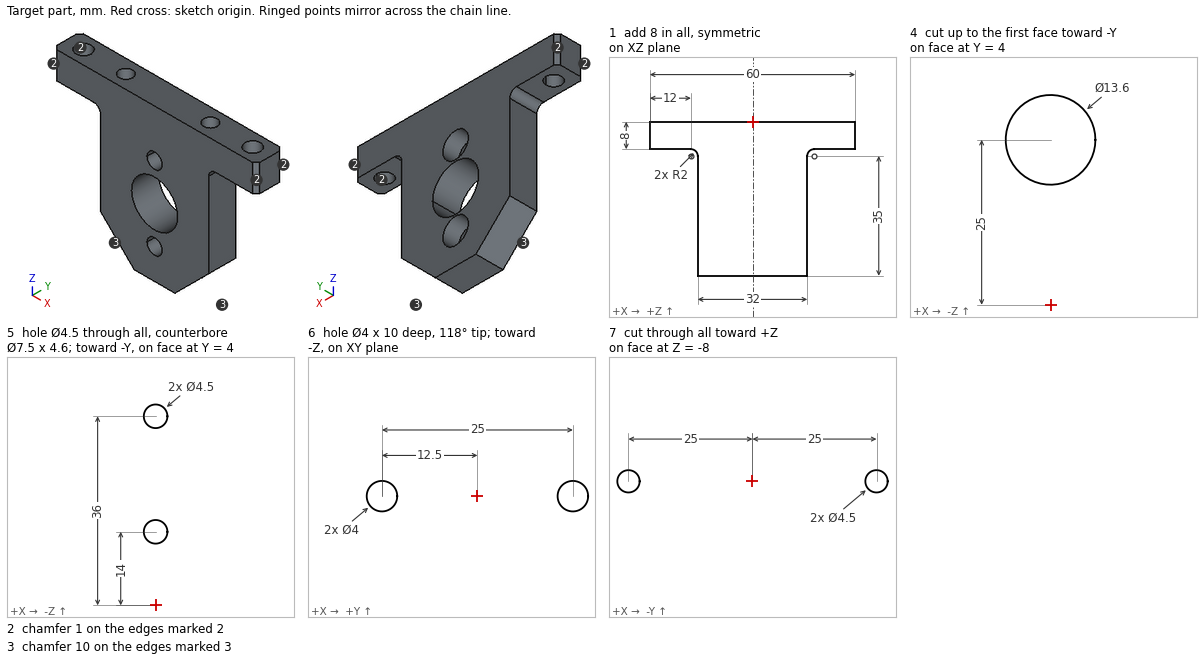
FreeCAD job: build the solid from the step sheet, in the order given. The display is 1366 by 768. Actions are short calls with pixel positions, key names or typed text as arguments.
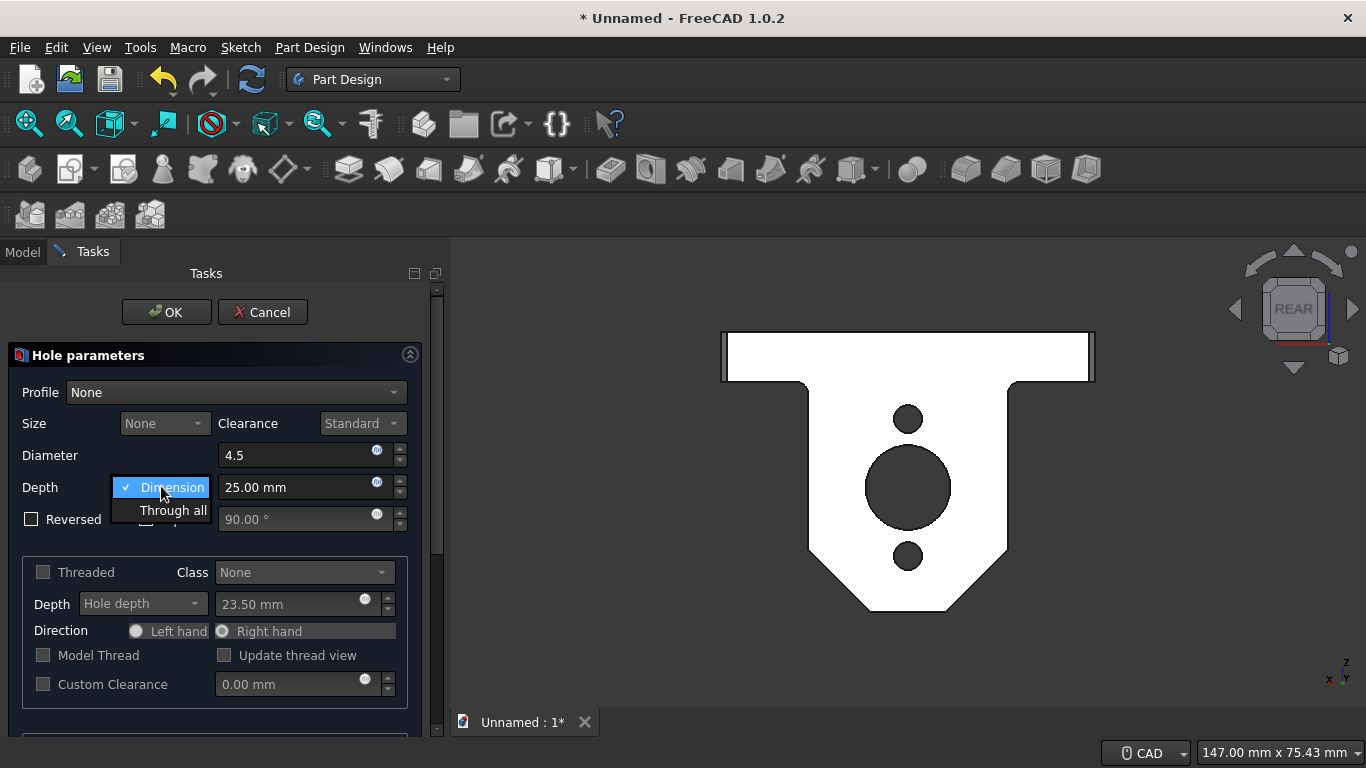
click(160, 510)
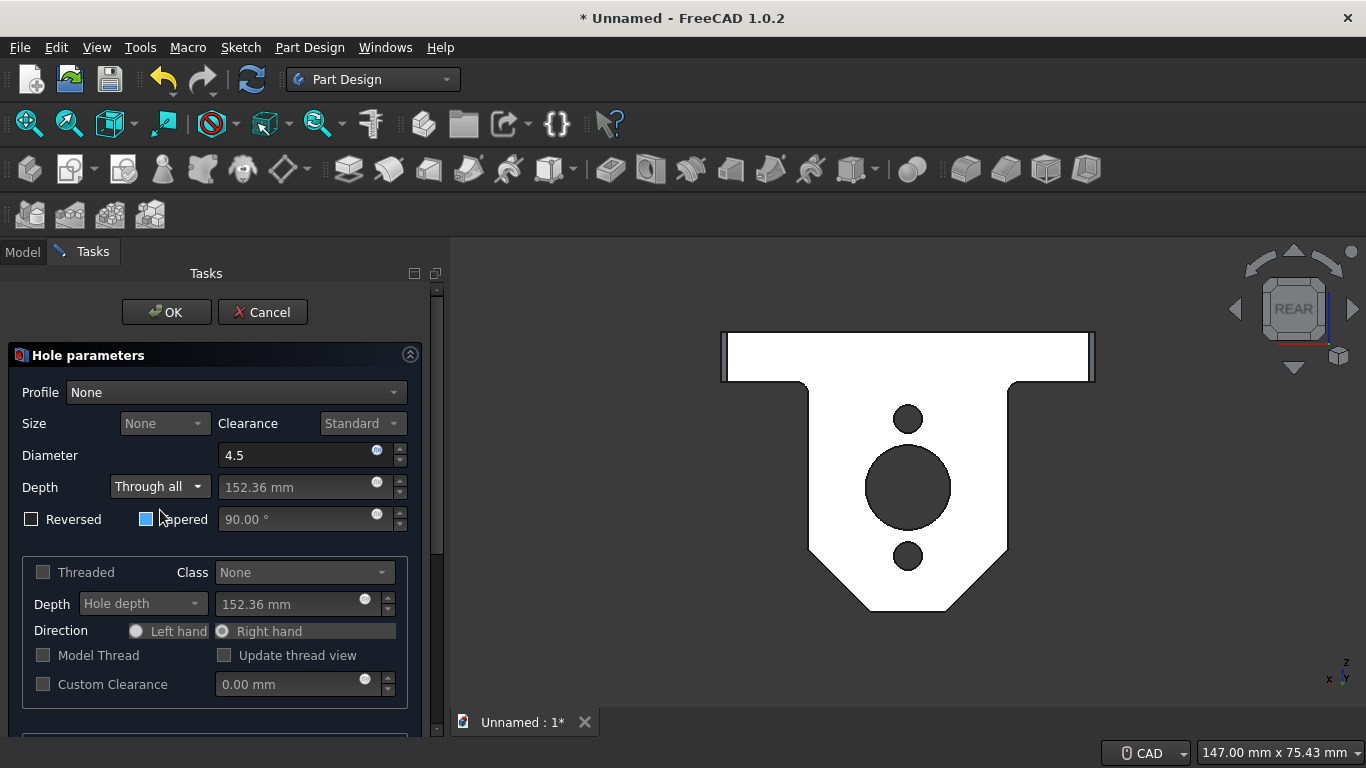
scroll(437, 510, down, 2)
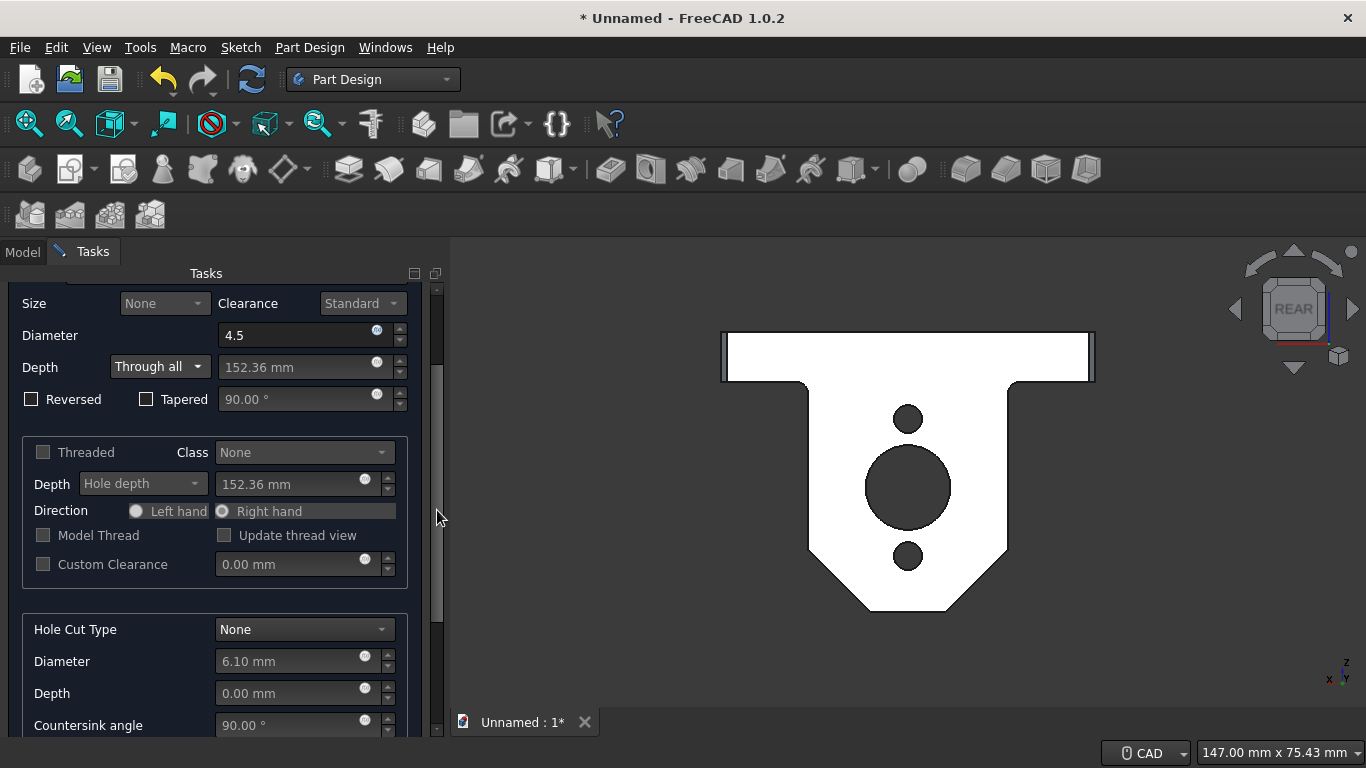
click(306, 630)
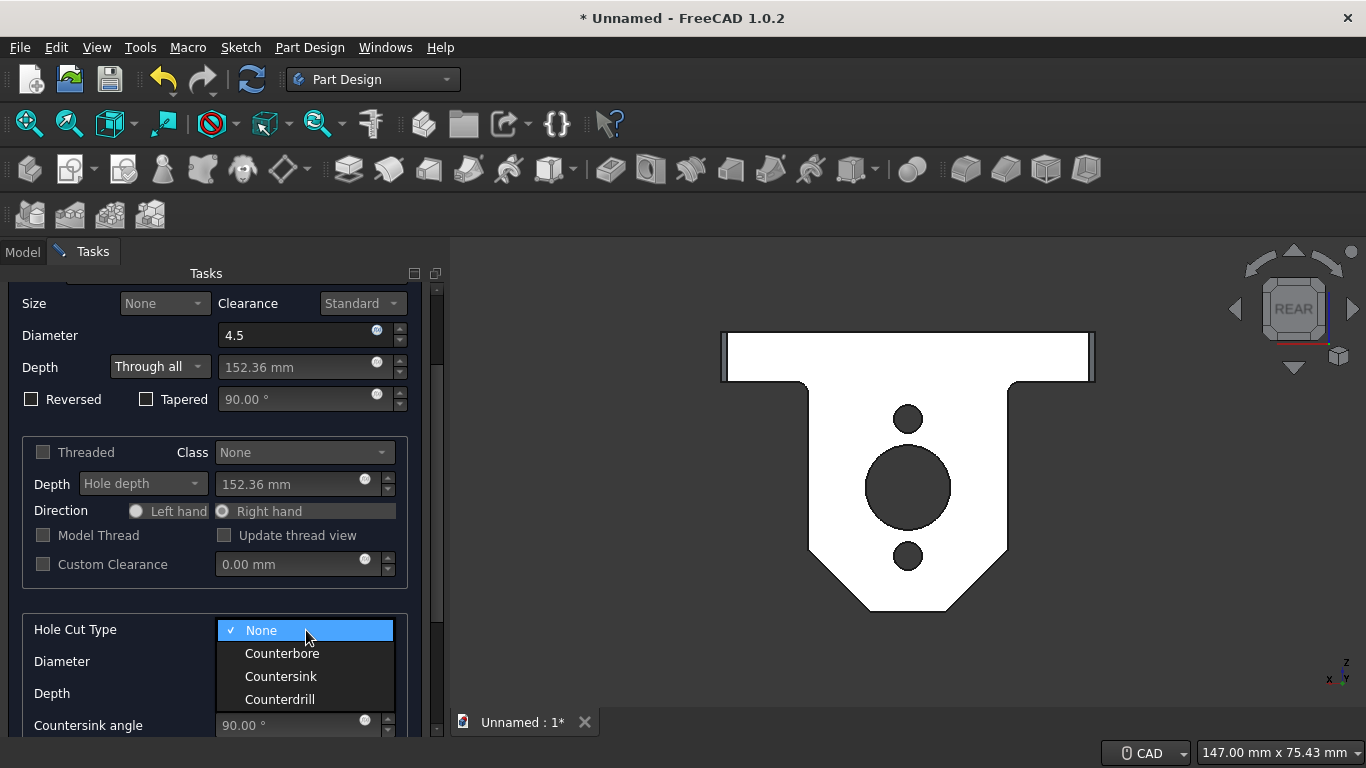
click(304, 654)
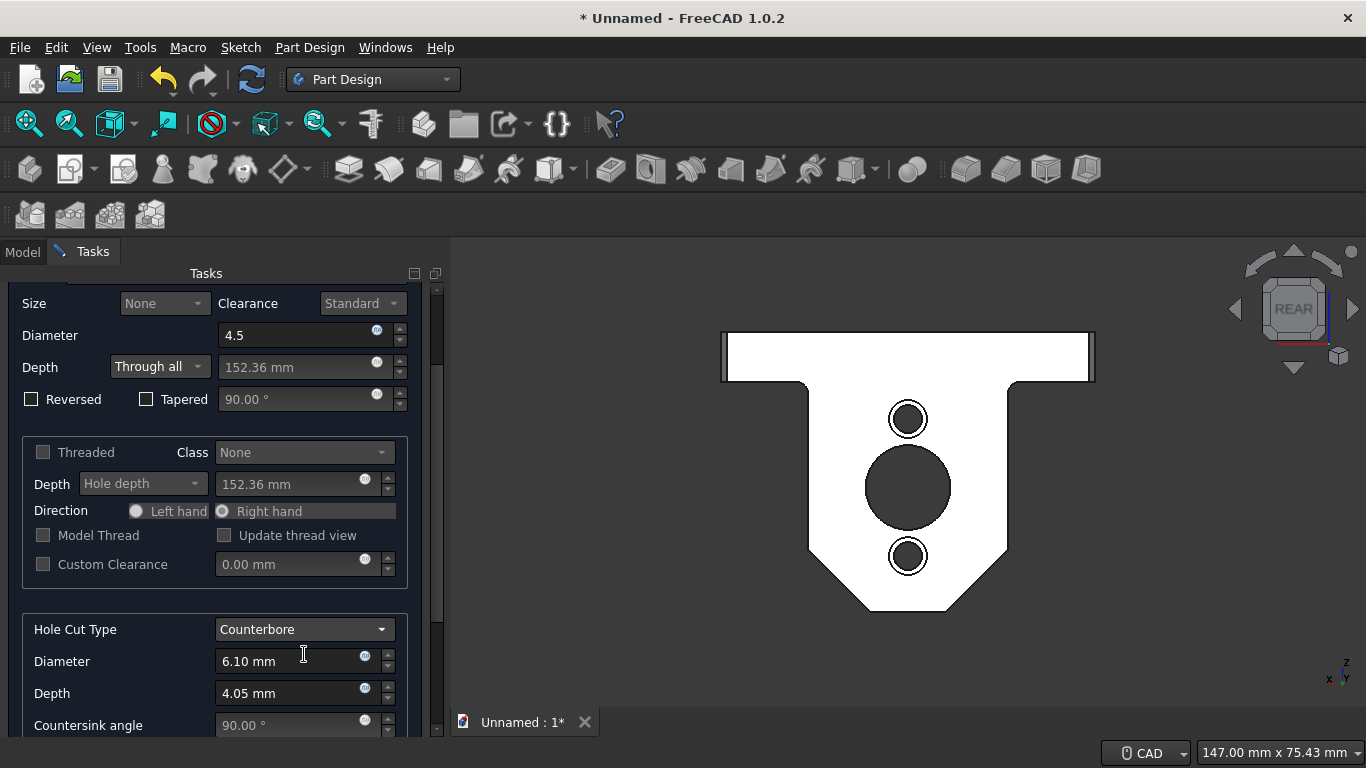
triple_click(298, 661)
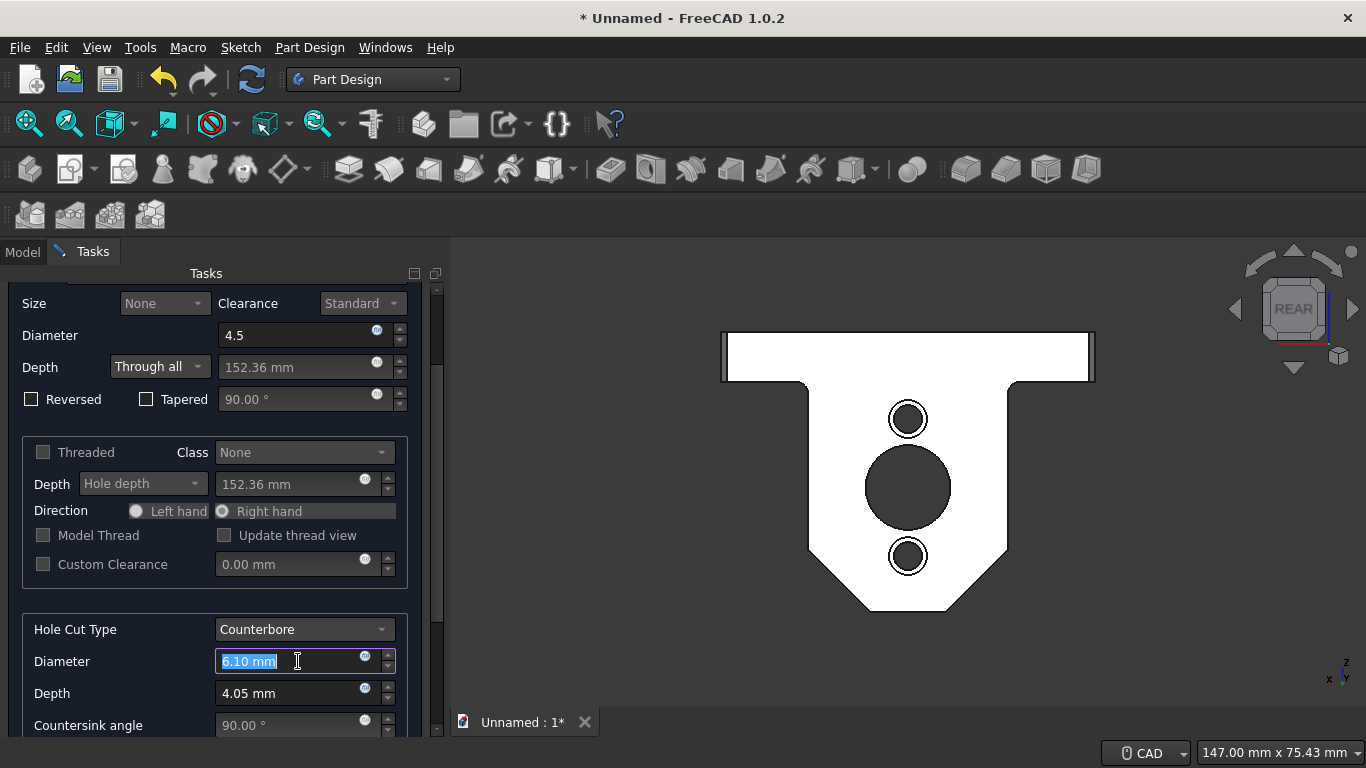
text(7.5)
key(Tab)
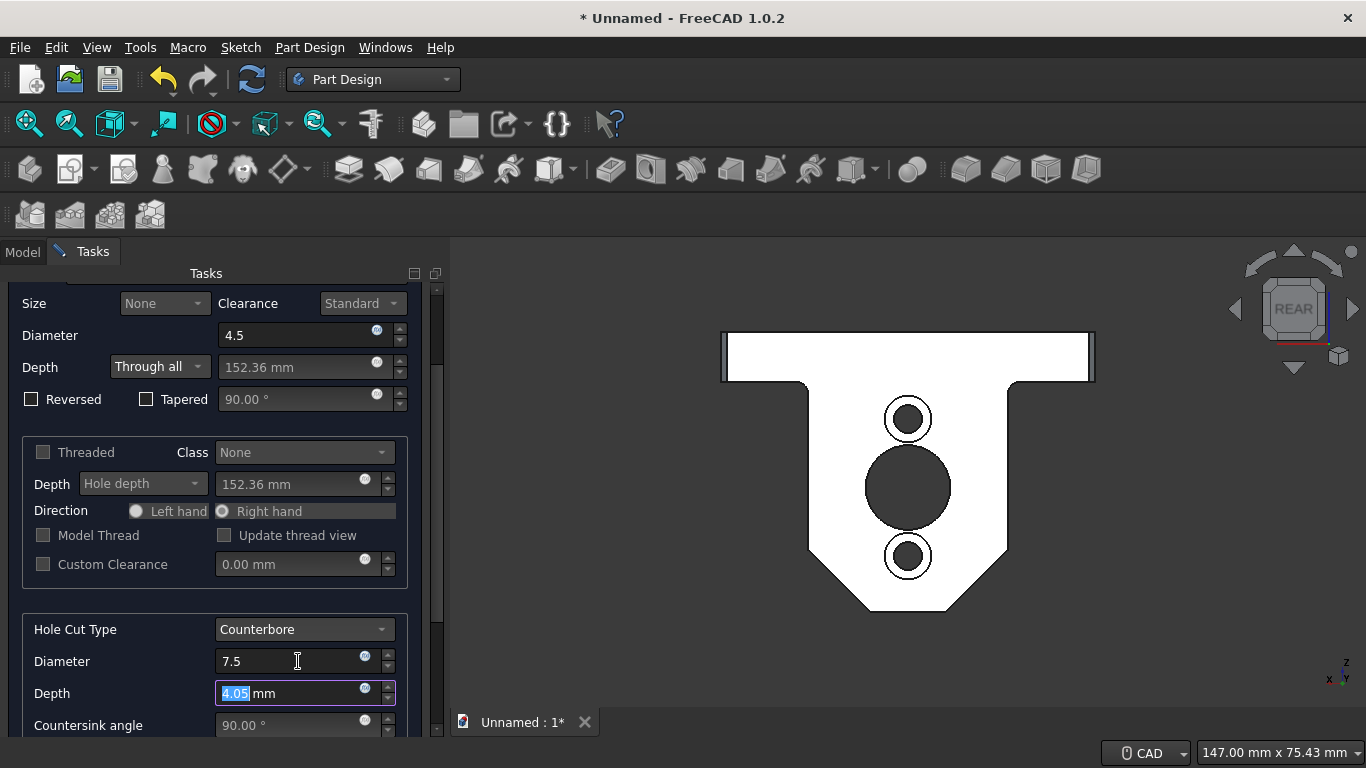
text(4.6)
key(Tab)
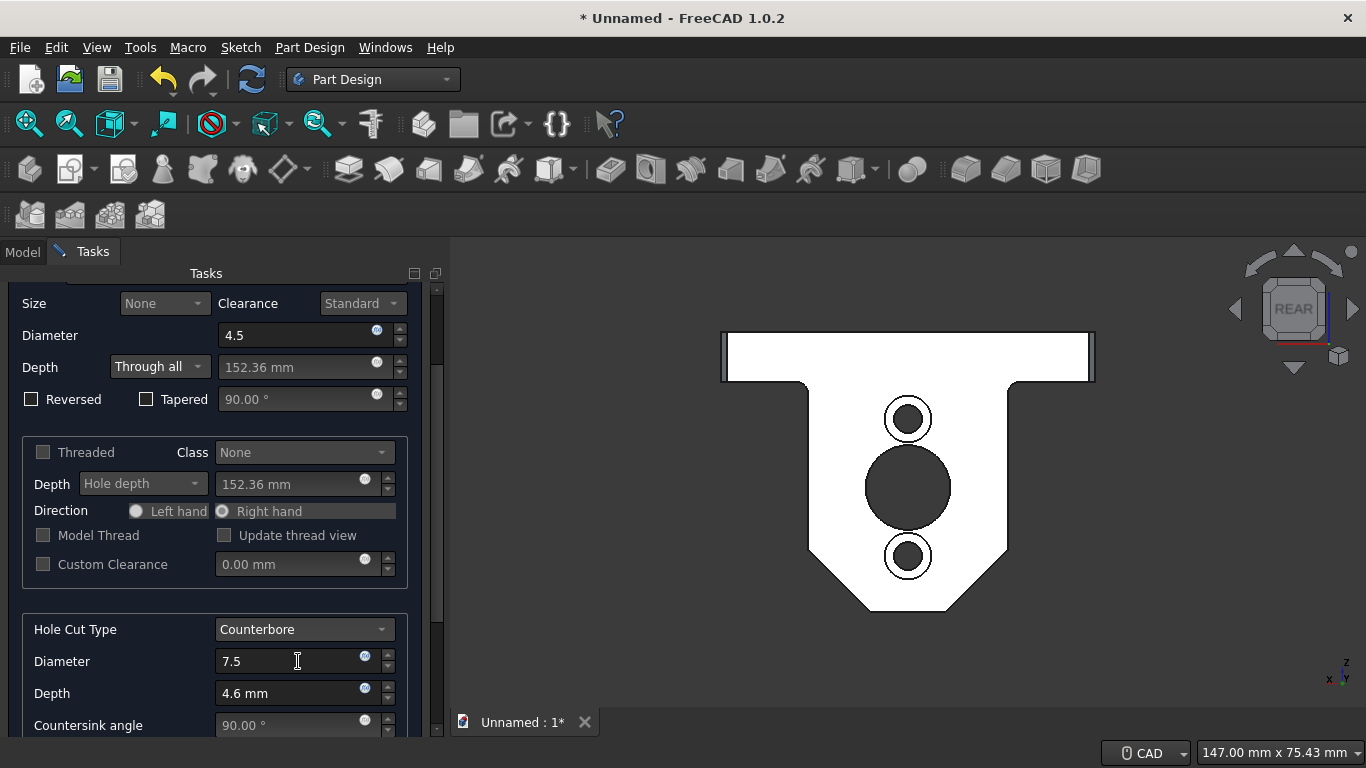
scroll(437, 510, up, 3)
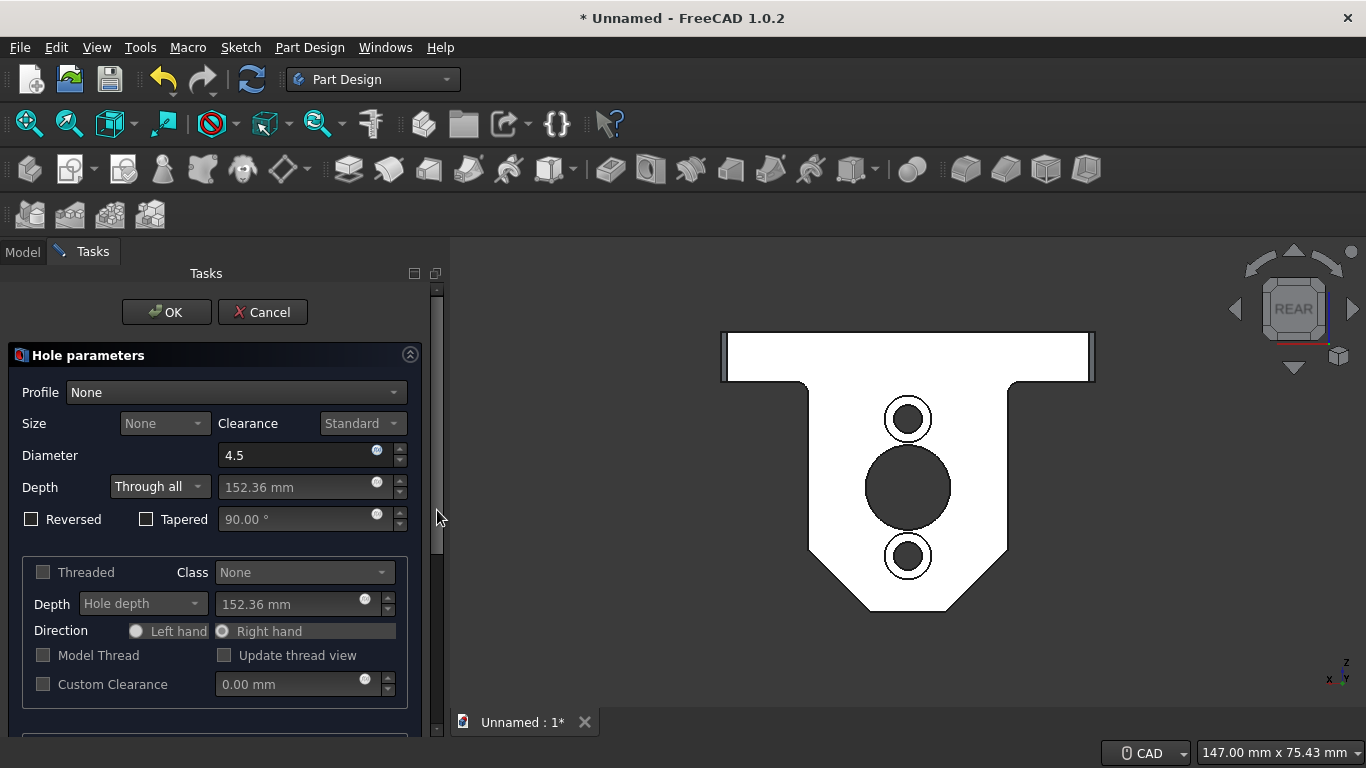
click(167, 312)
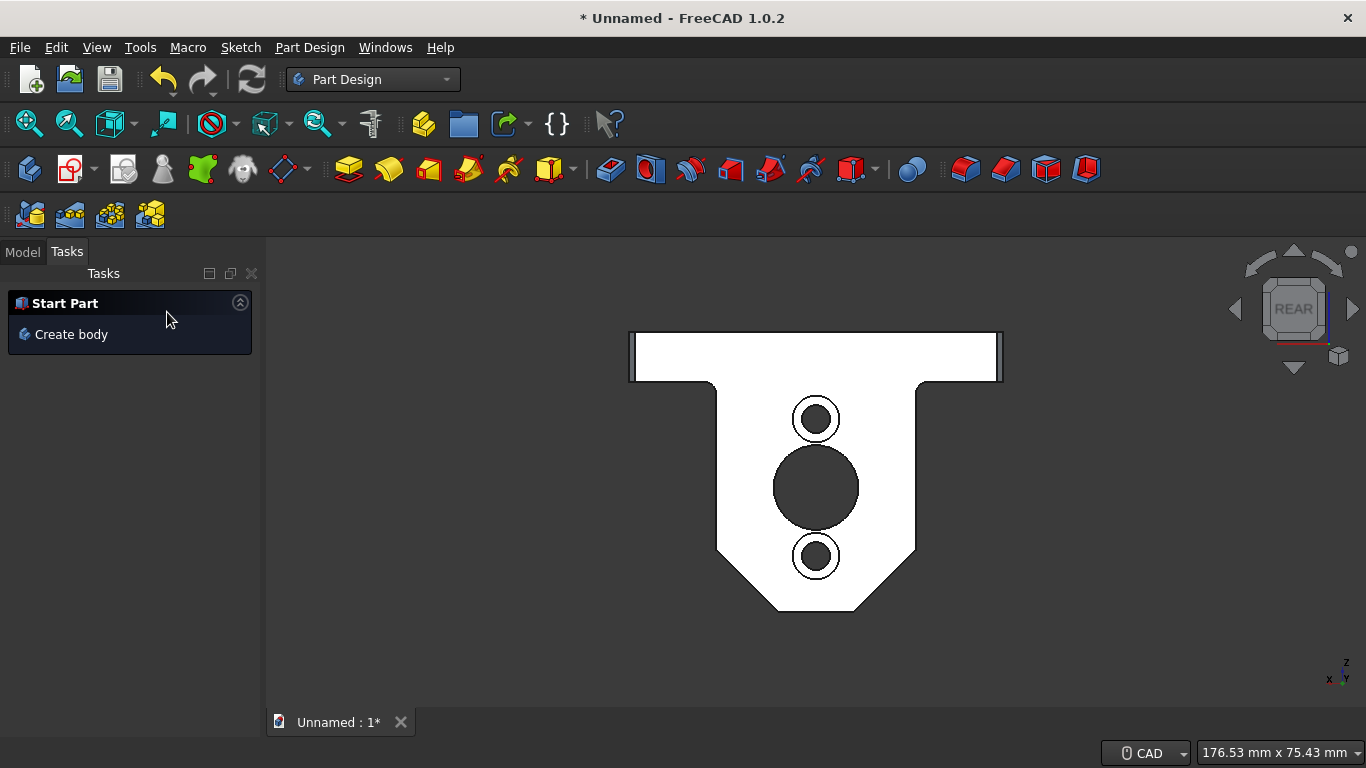
click(70, 170)